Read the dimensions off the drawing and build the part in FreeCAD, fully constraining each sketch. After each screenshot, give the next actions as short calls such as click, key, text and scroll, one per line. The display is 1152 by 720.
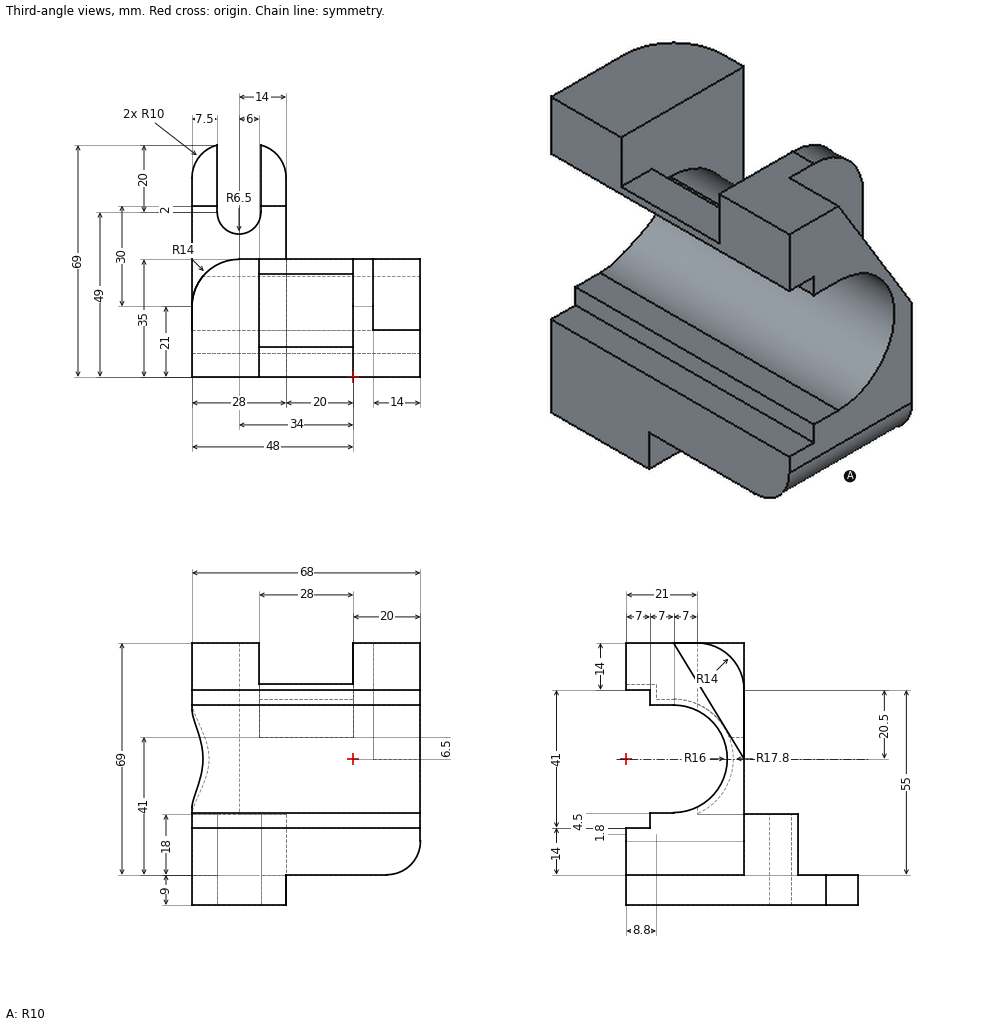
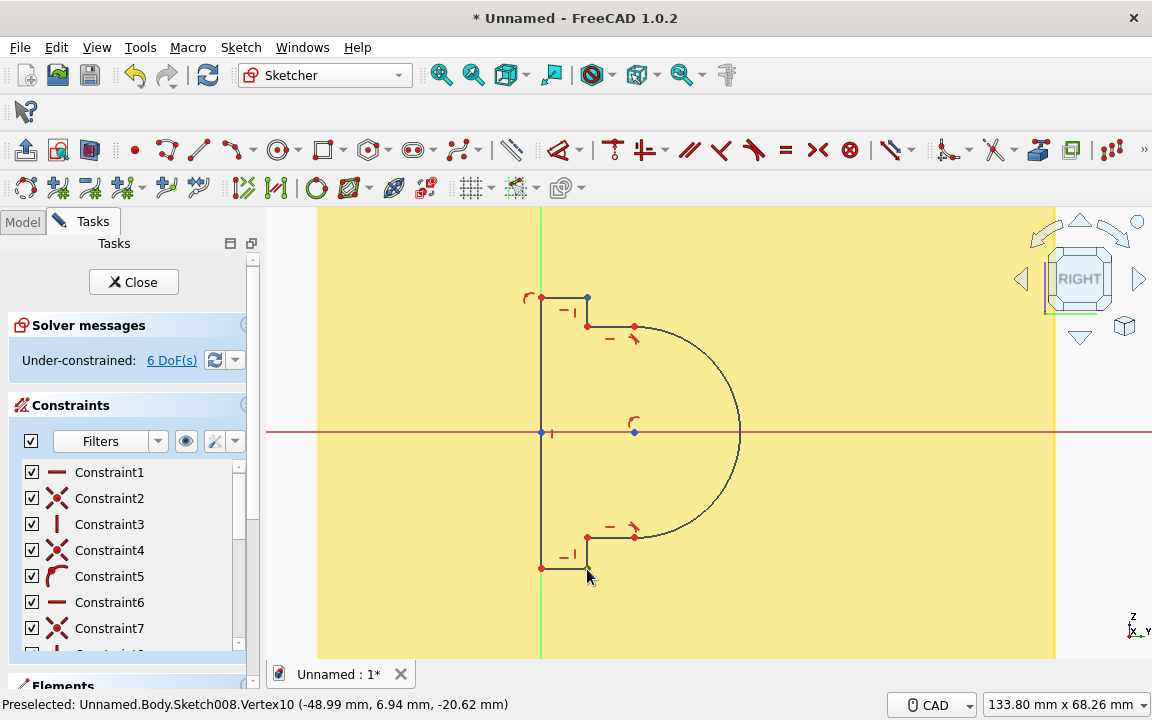
click(344, 432)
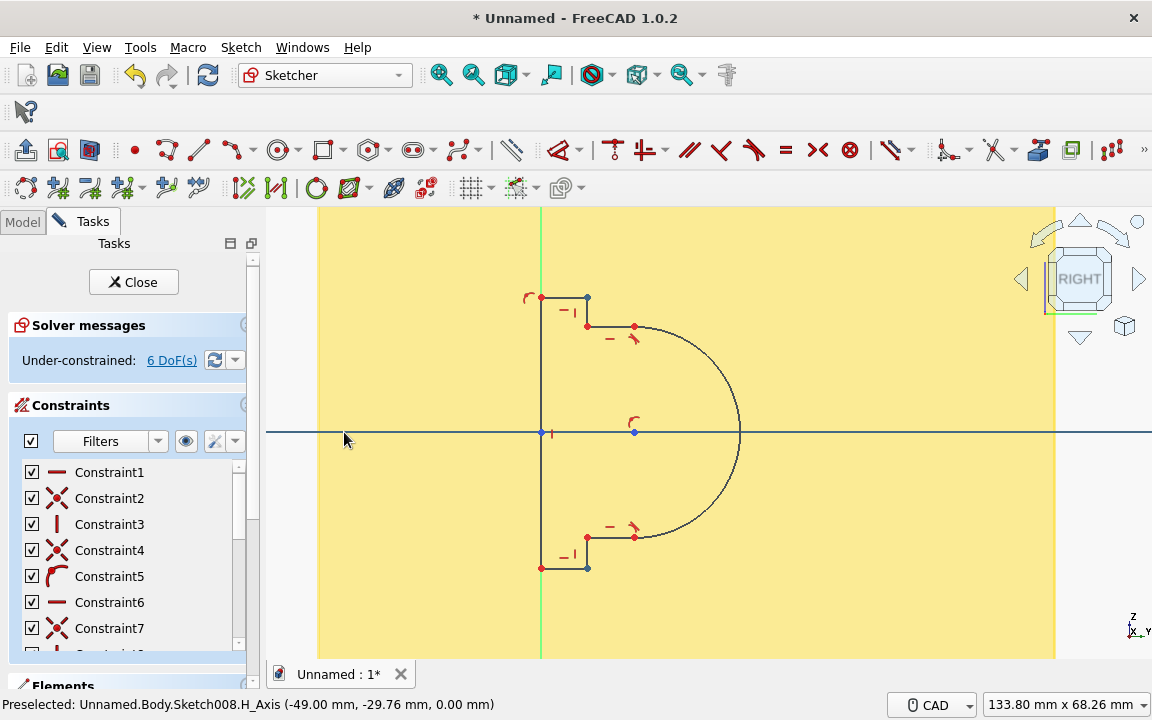
click(818, 150)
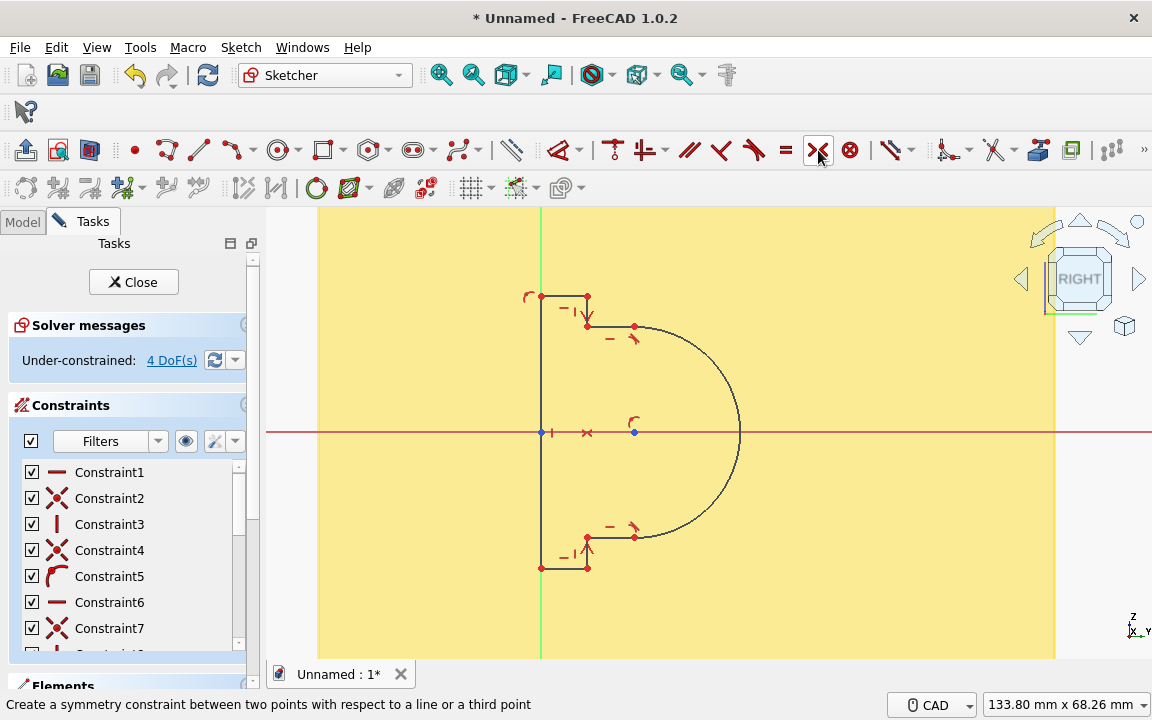
click(558, 150)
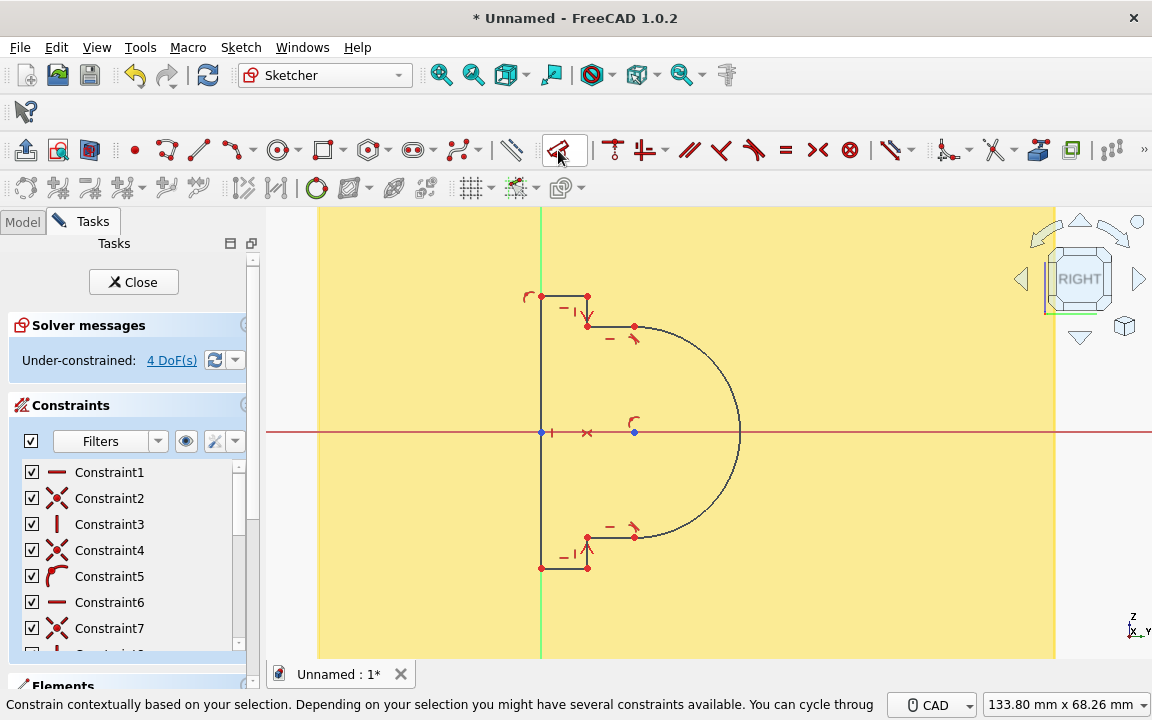
click(720, 494)
click(746, 513)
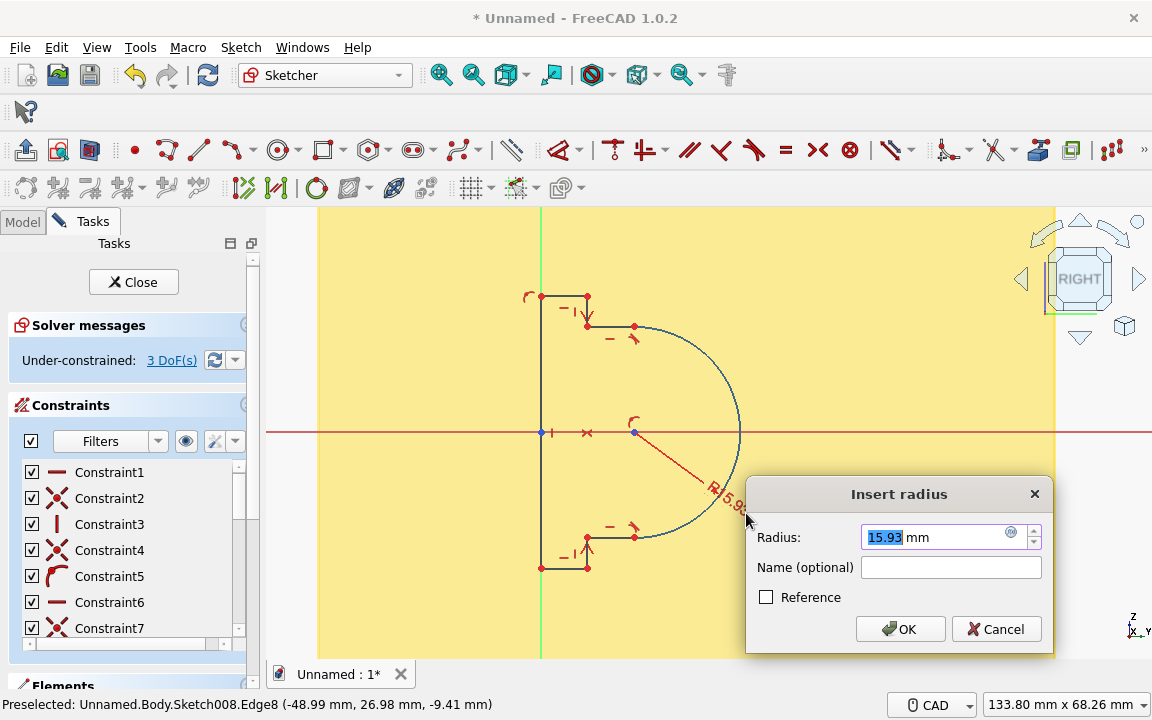
text(16)
key(Return)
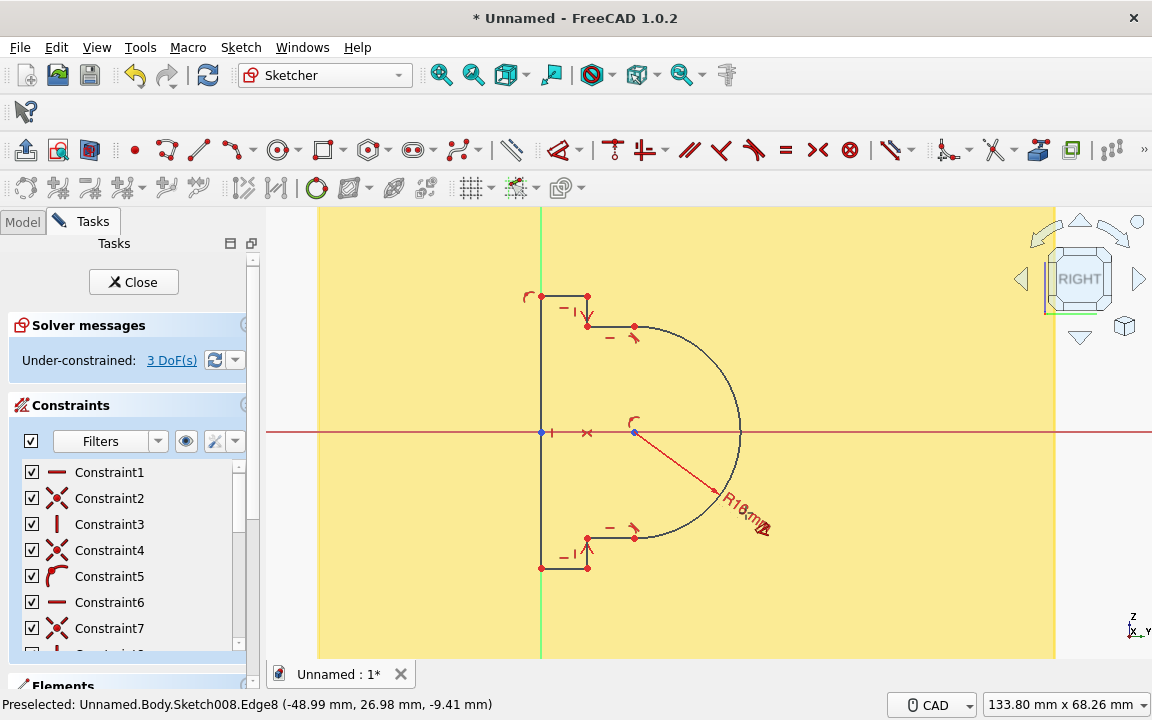
click(620, 327)
click(611, 293)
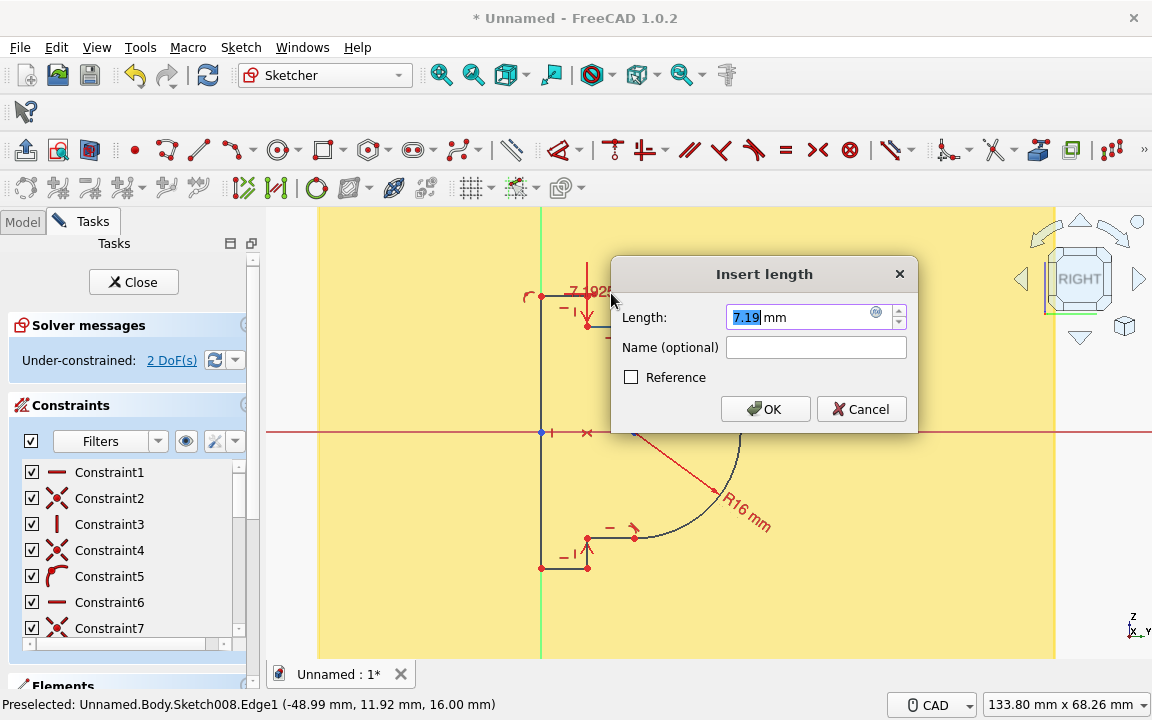
text(7)
key(Return)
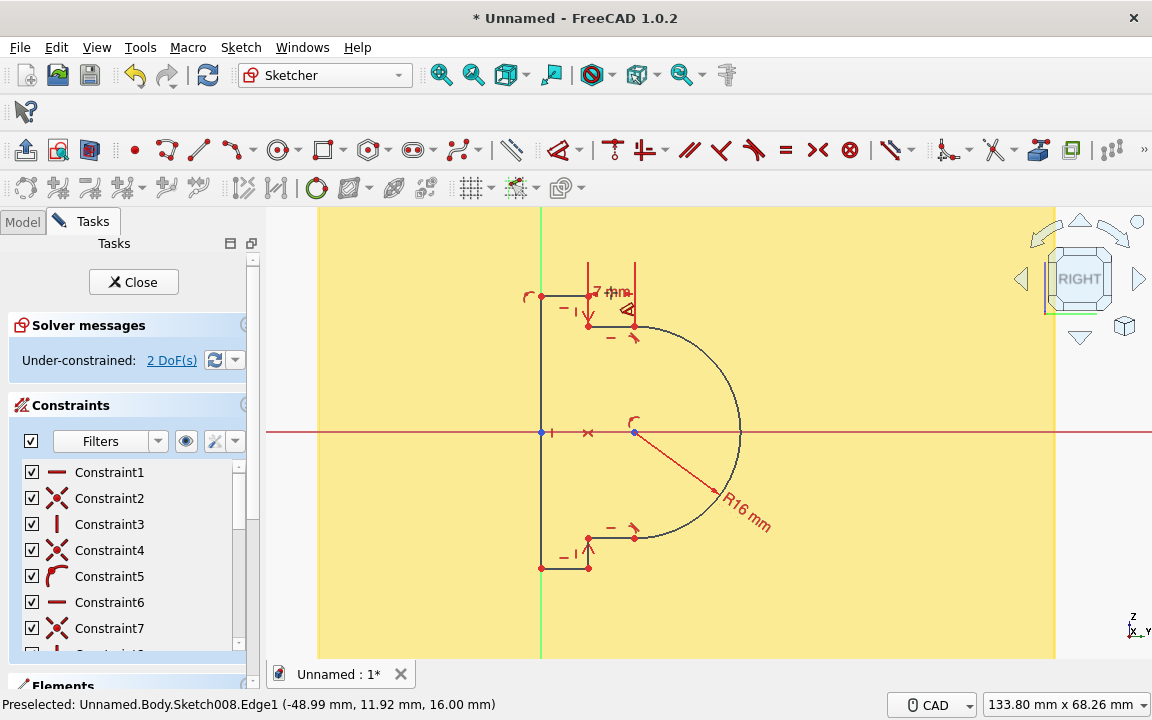
click(574, 296)
click(565, 262)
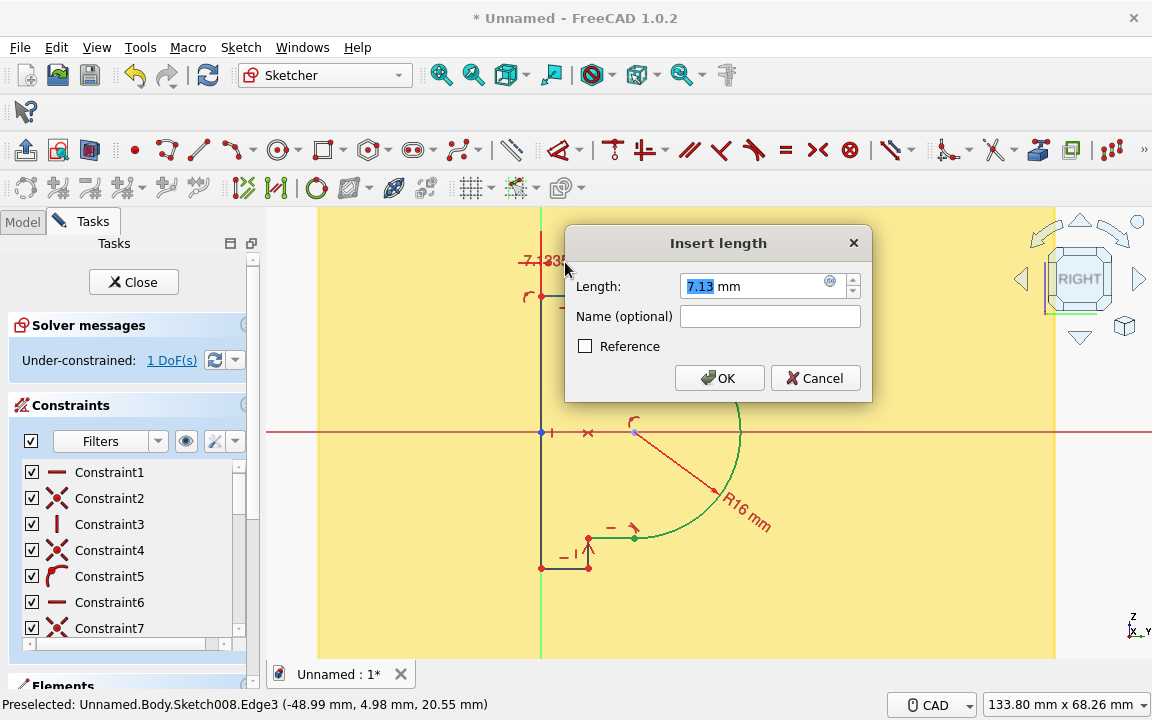
text(7)
key(Return)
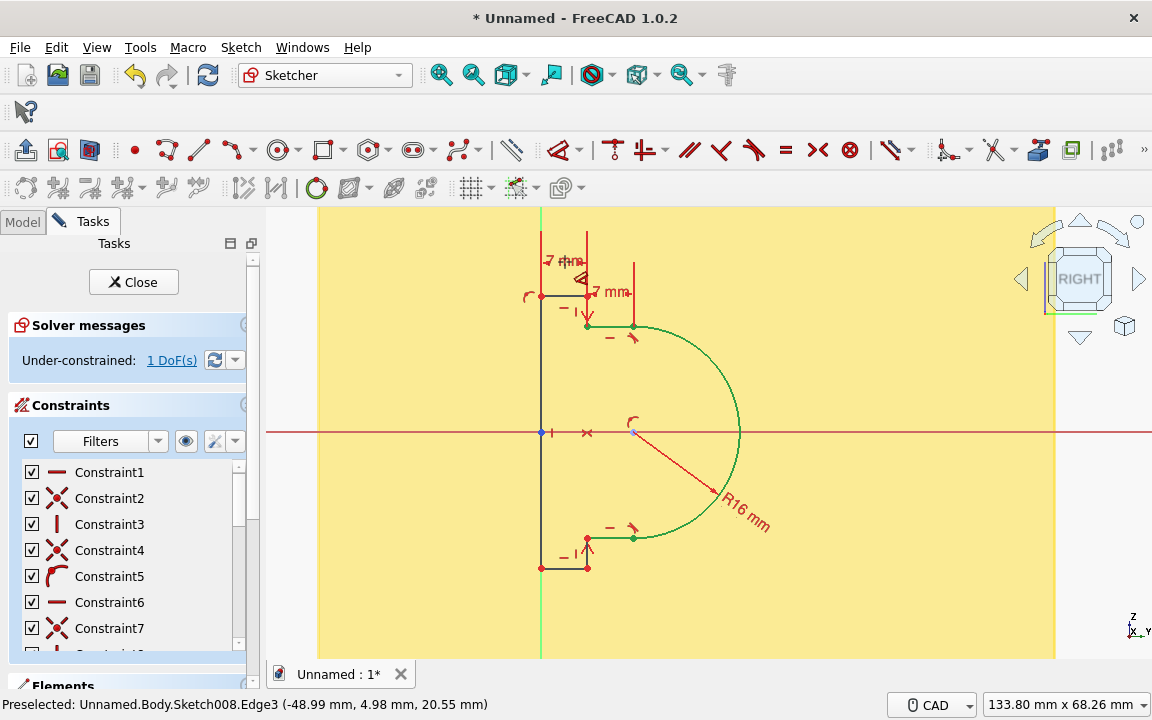
click(541, 378)
click(507, 370)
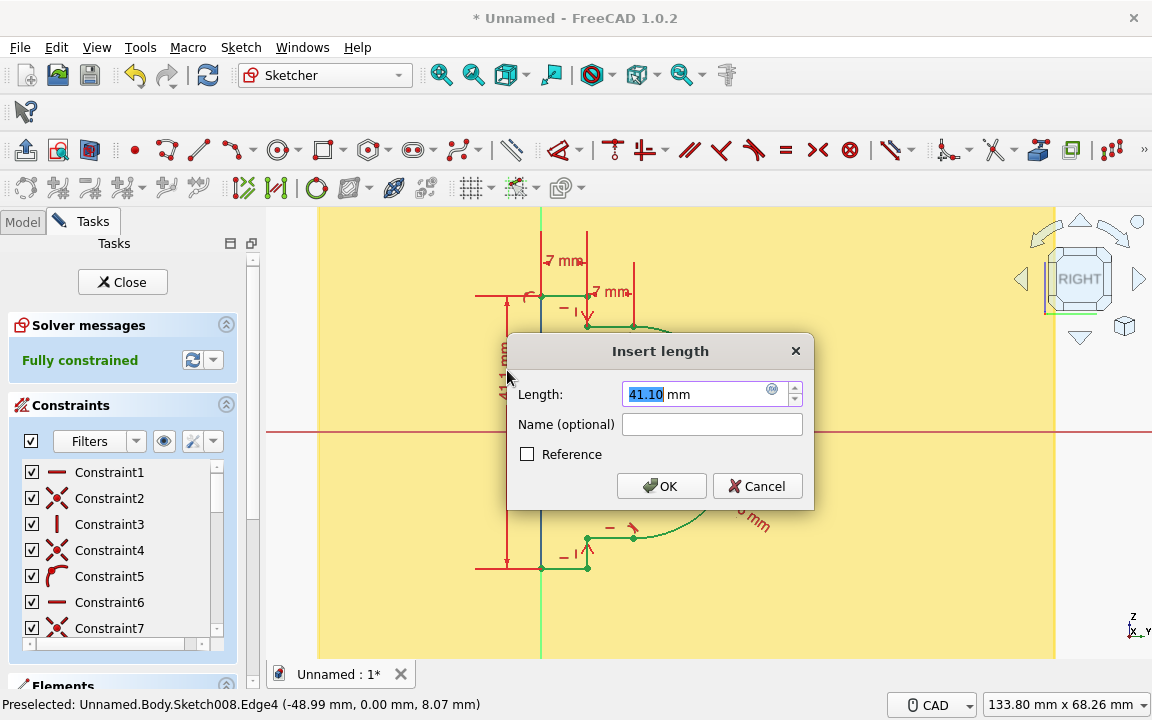
text(41)
key(Return)
key(Escape)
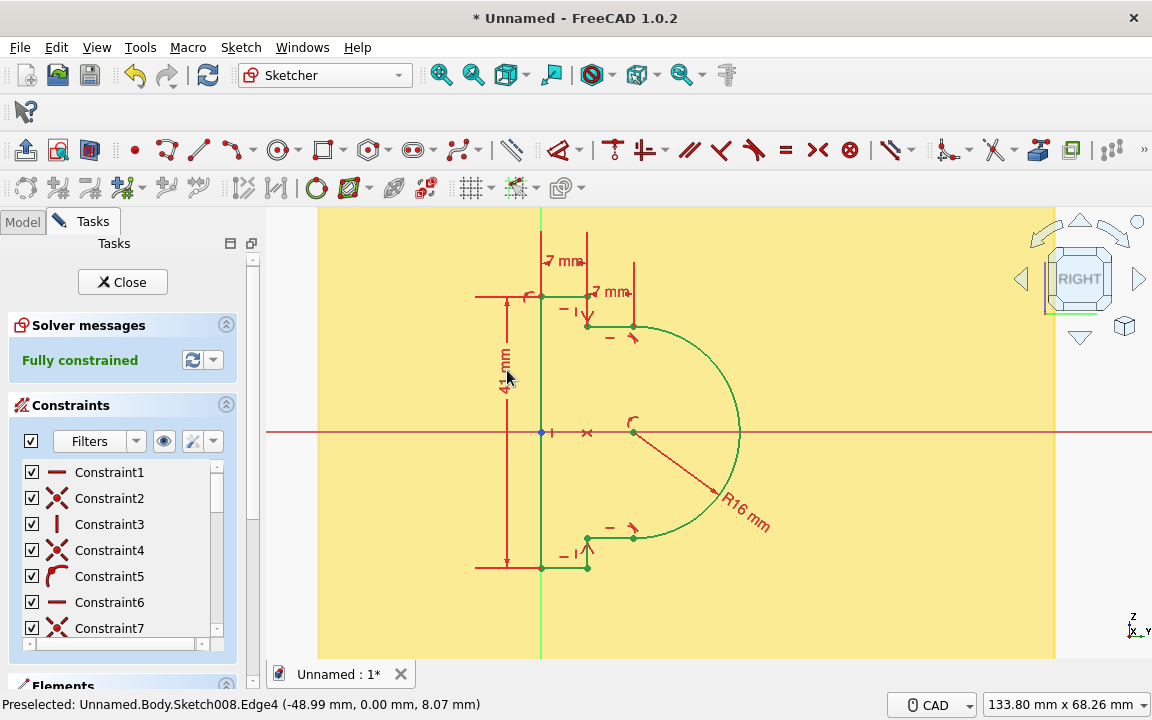
click(123, 282)